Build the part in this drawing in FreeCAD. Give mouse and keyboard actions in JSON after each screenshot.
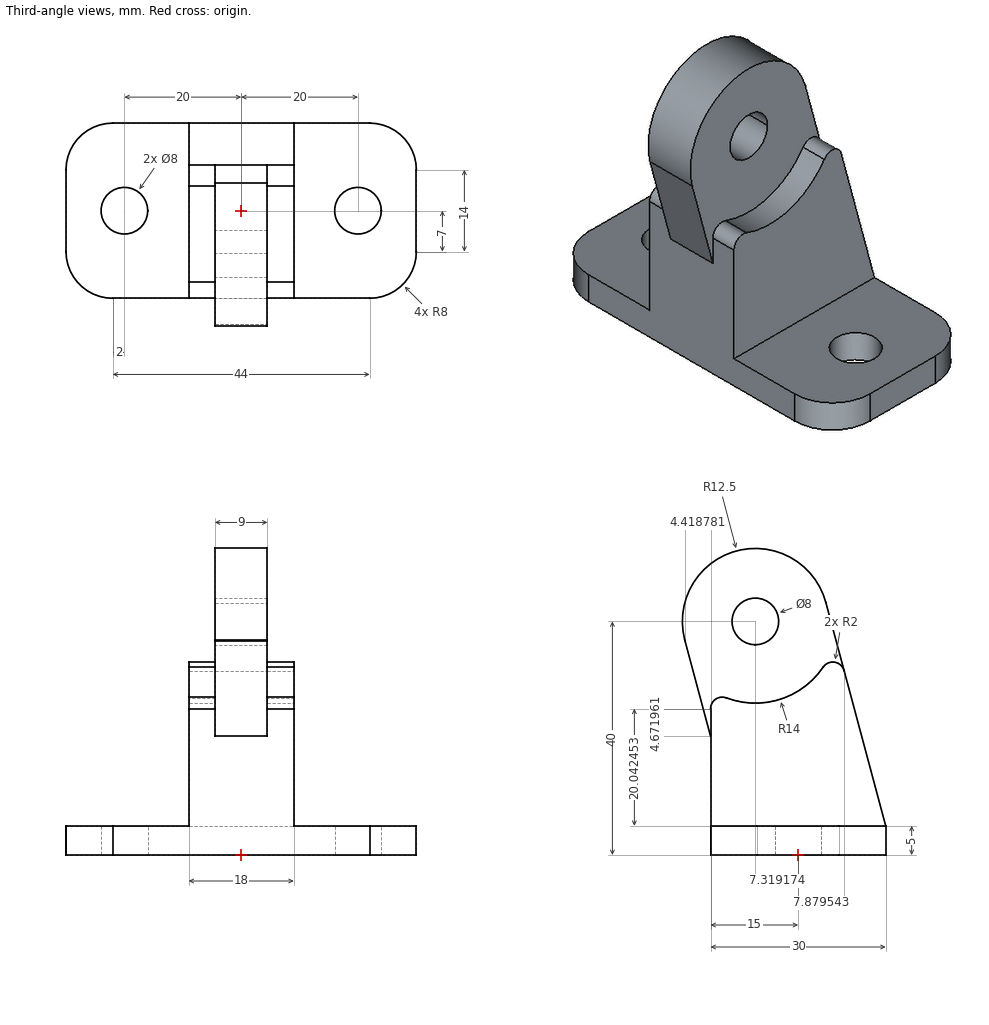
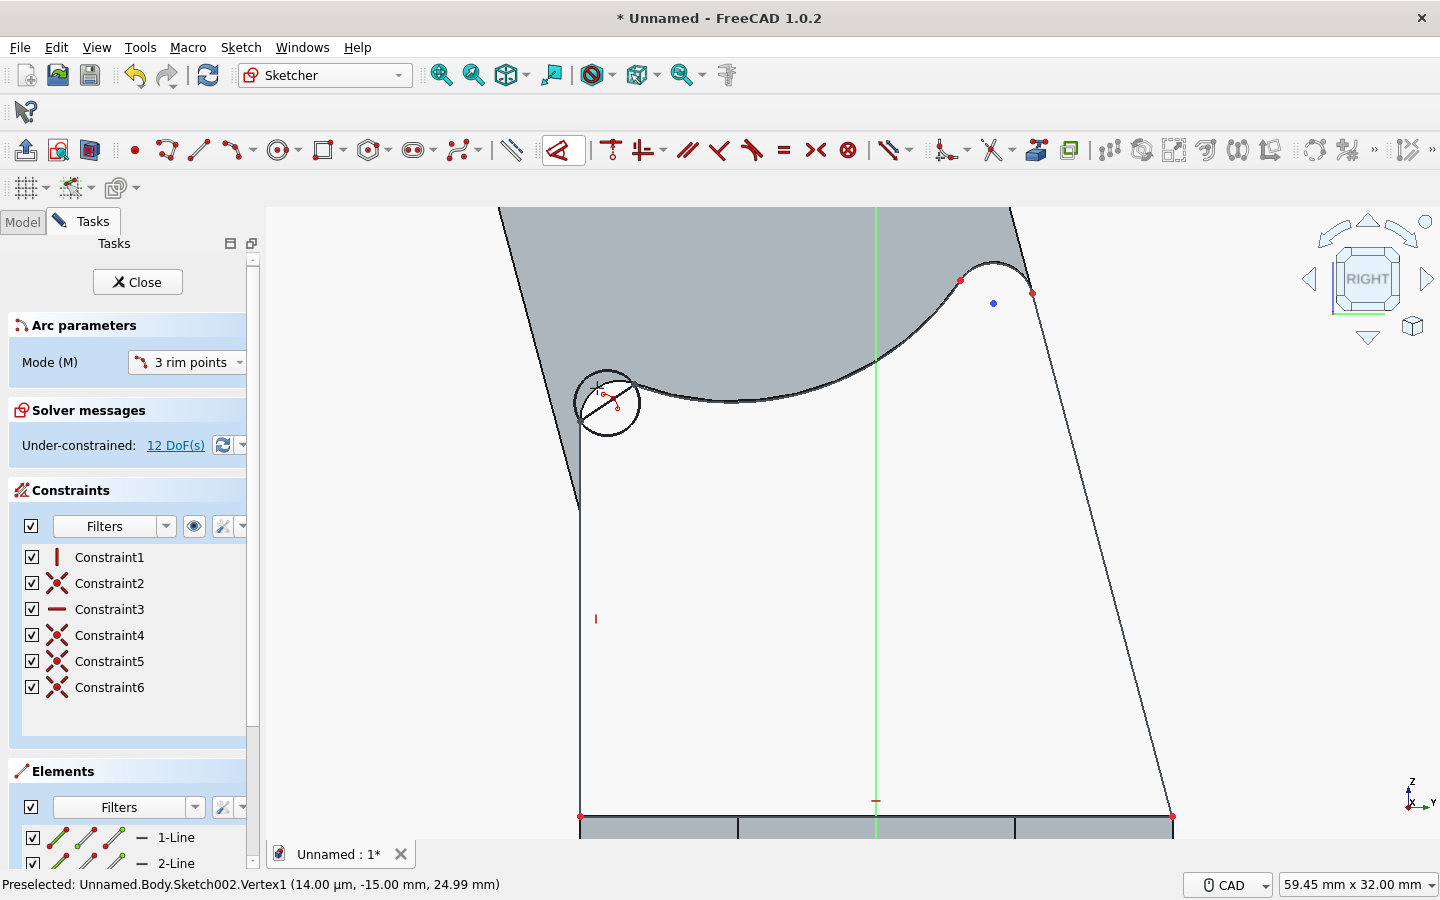
{"action": "left_click", "coordinate": [597, 388]}
{"action": "key", "text": "Escape"}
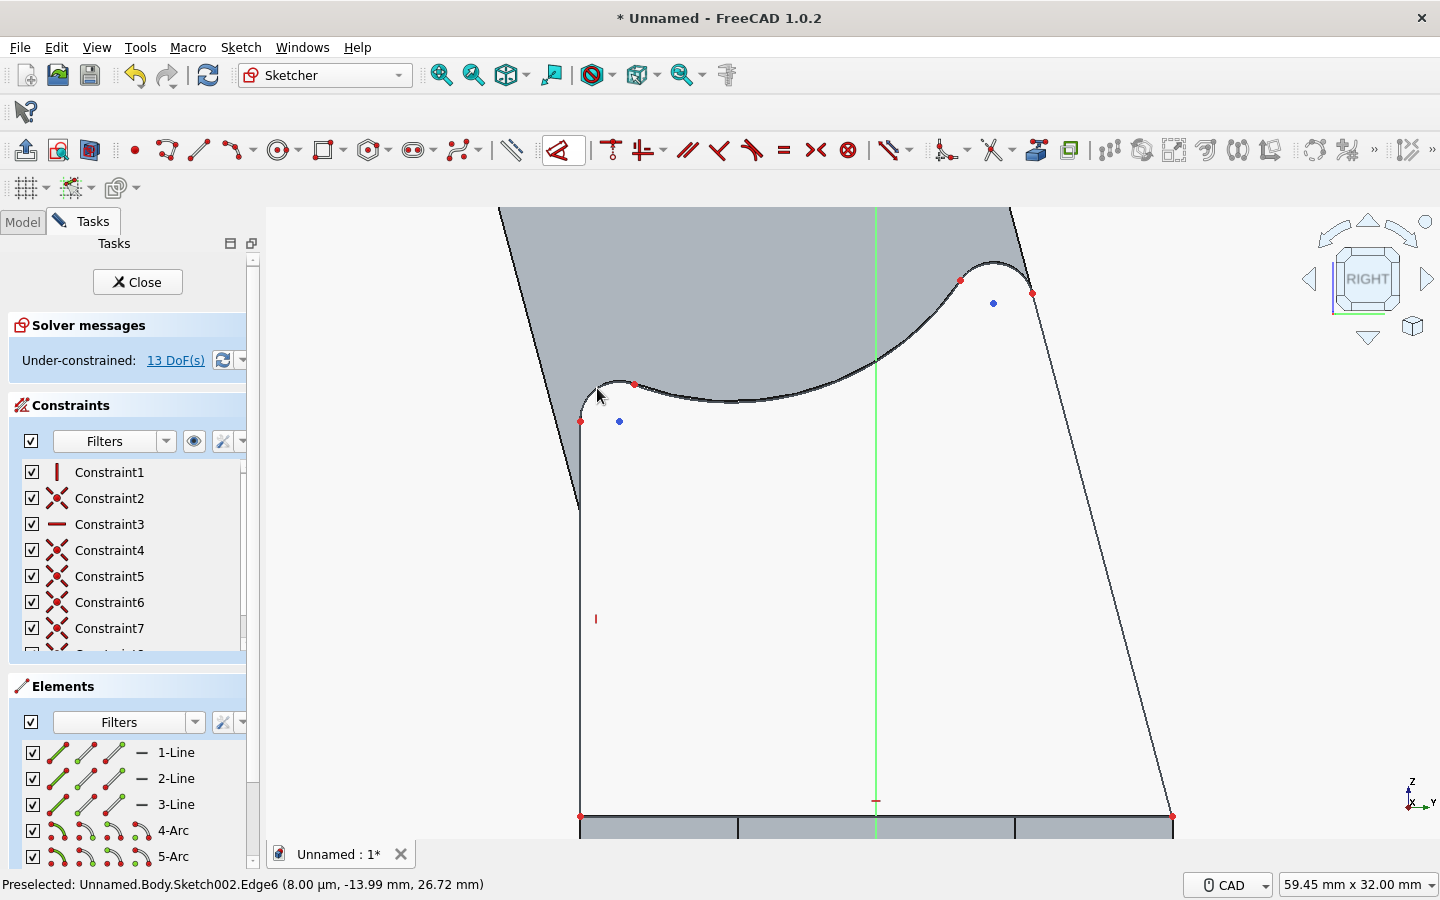
{"action": "left_click", "coordinate": [580, 540]}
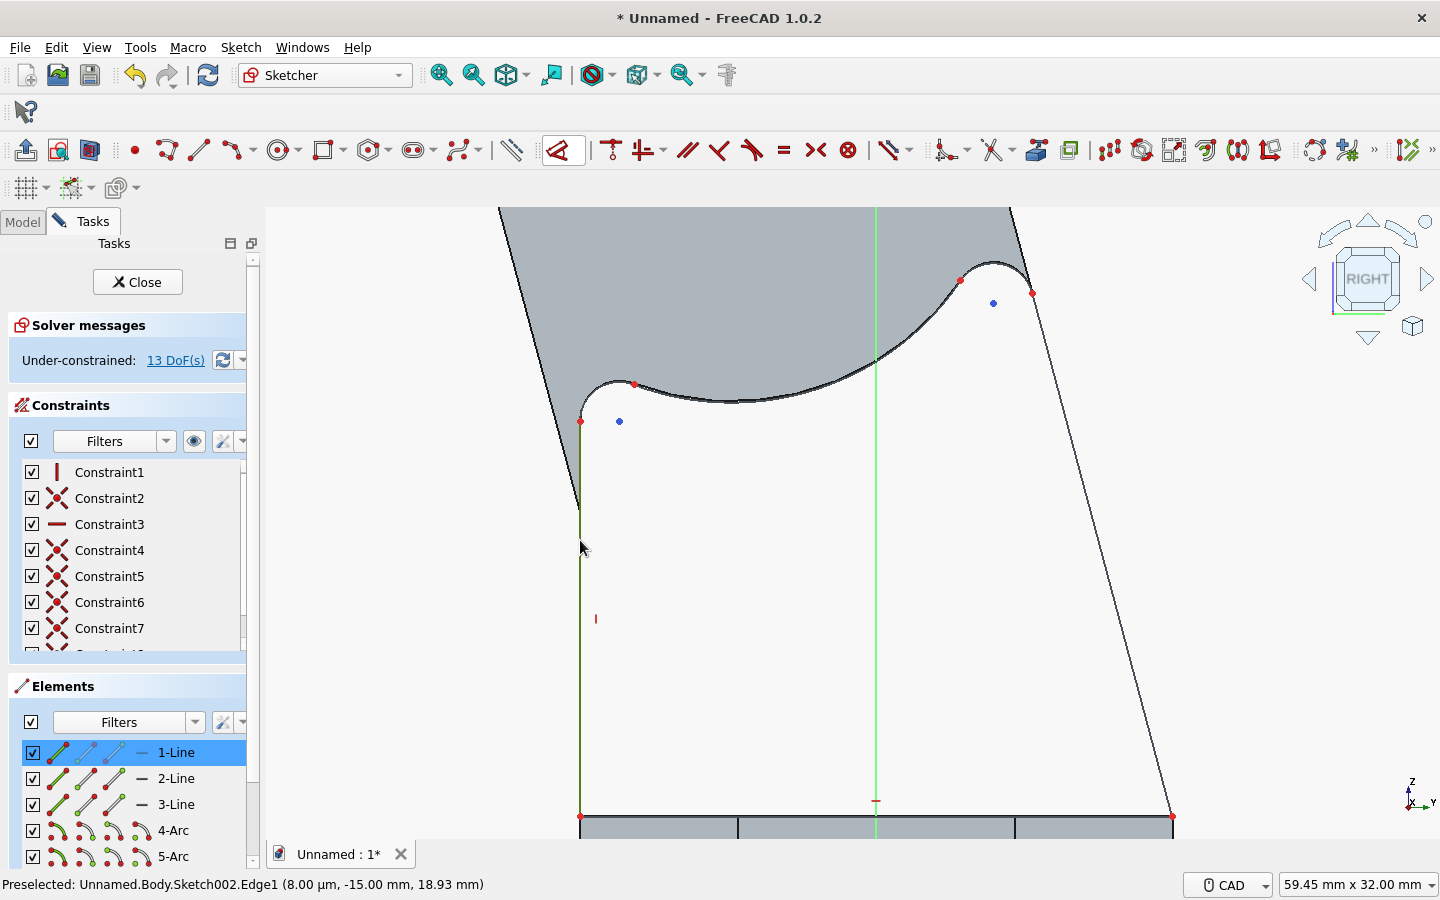
{"action": "left_click", "coordinate": [612, 383]}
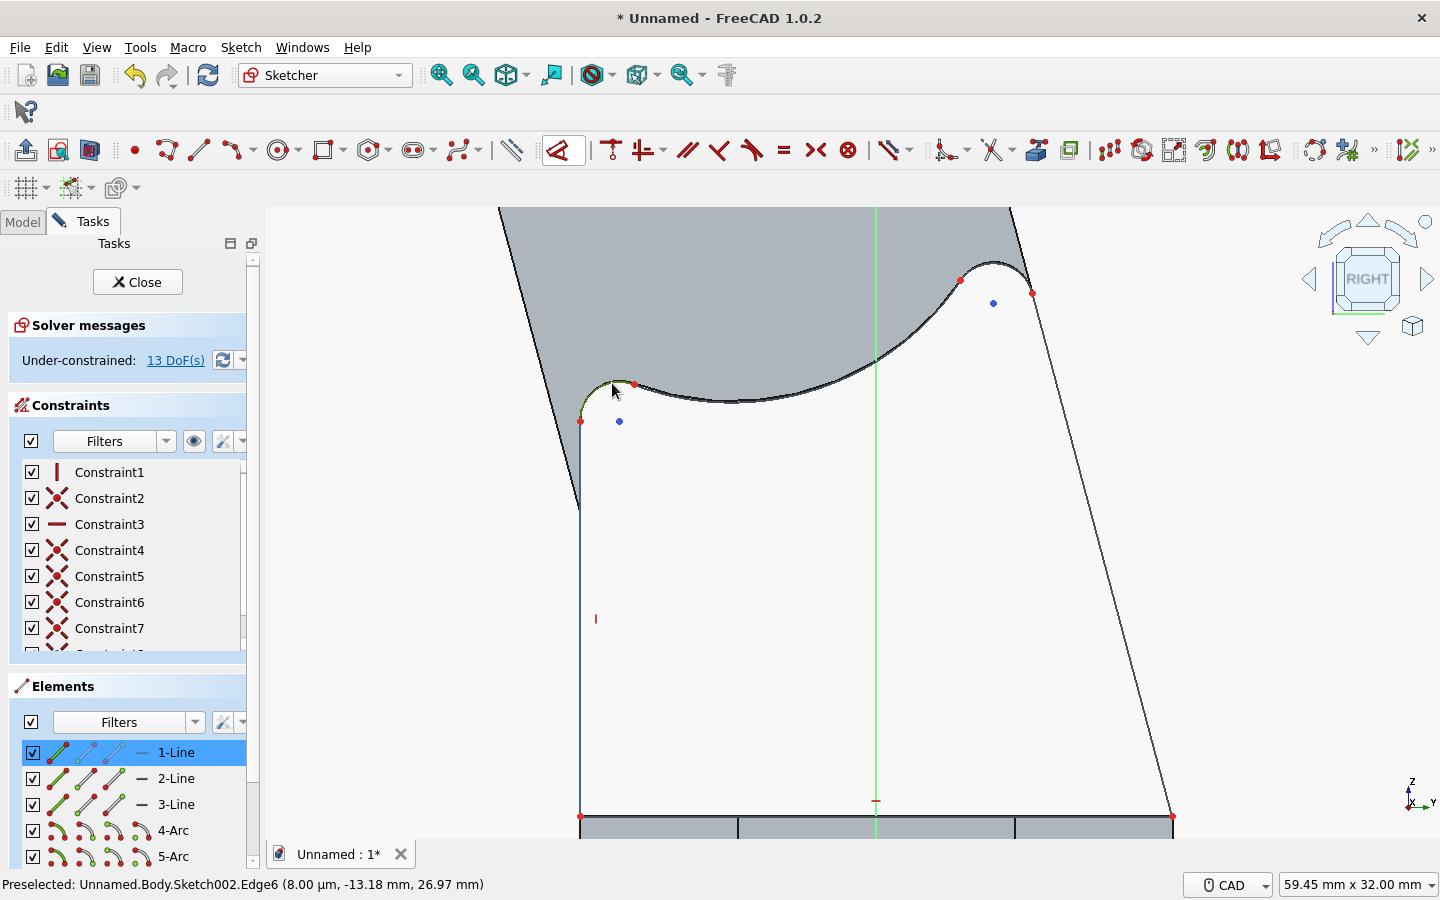
{"action": "left_click", "coordinate": [752, 150]}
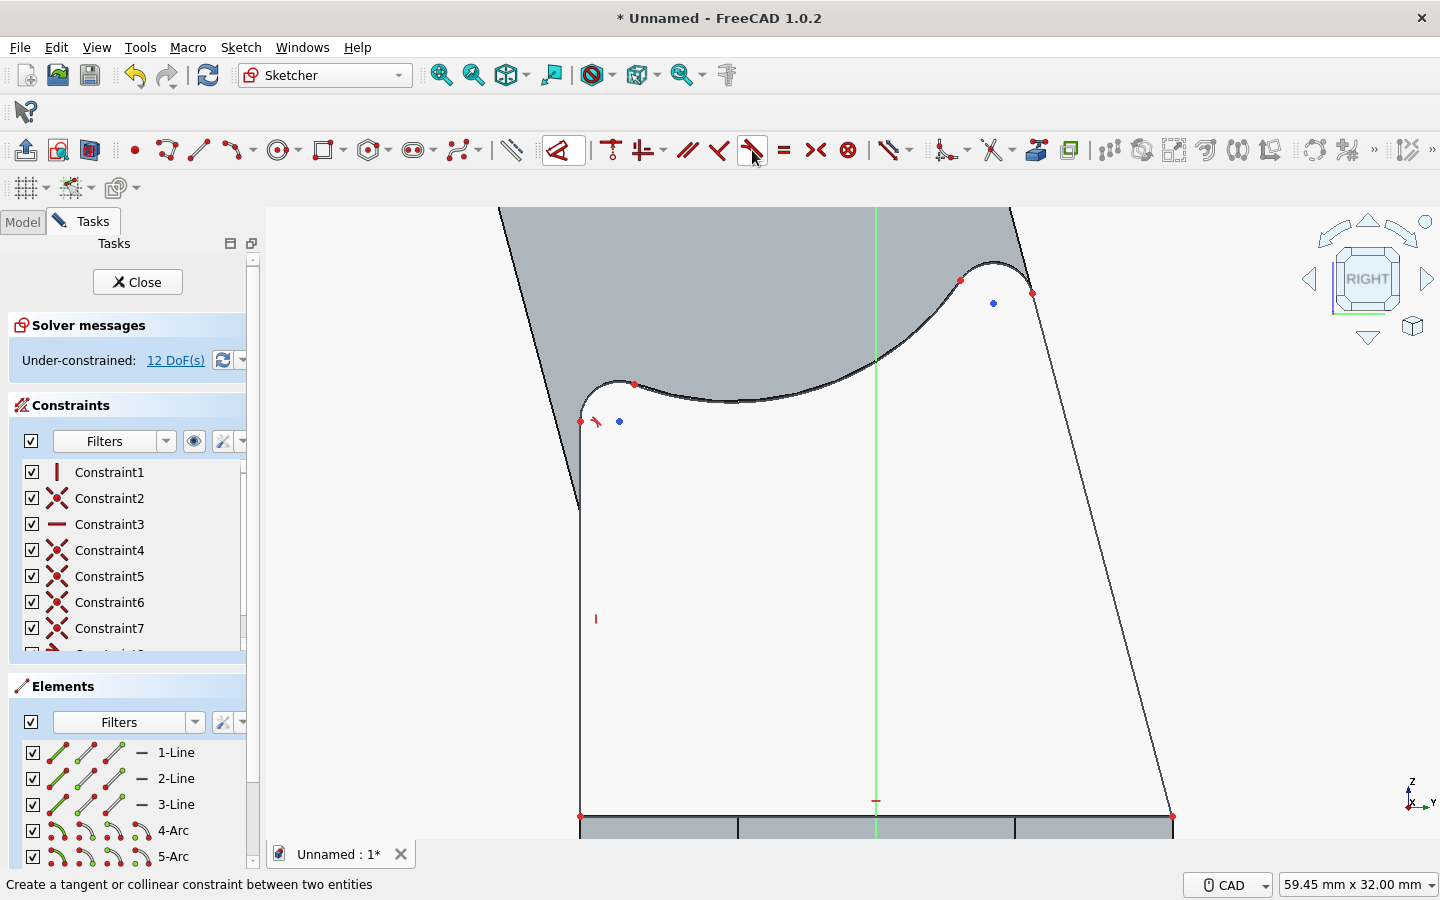
{"action": "left_click", "coordinate": [1130, 660]}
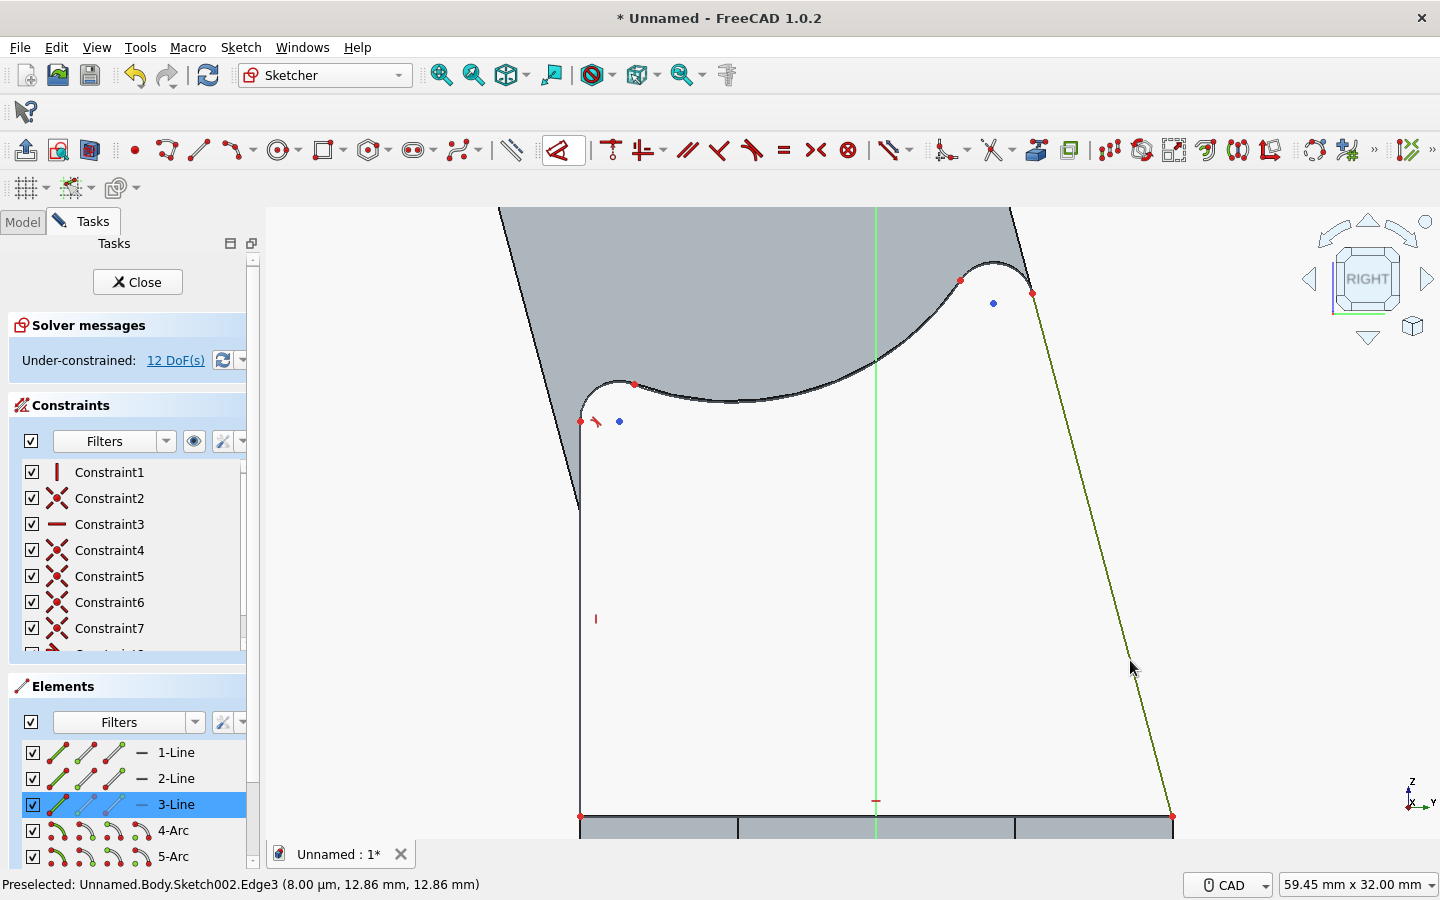
{"action": "left_click", "coordinate": [1017, 271]}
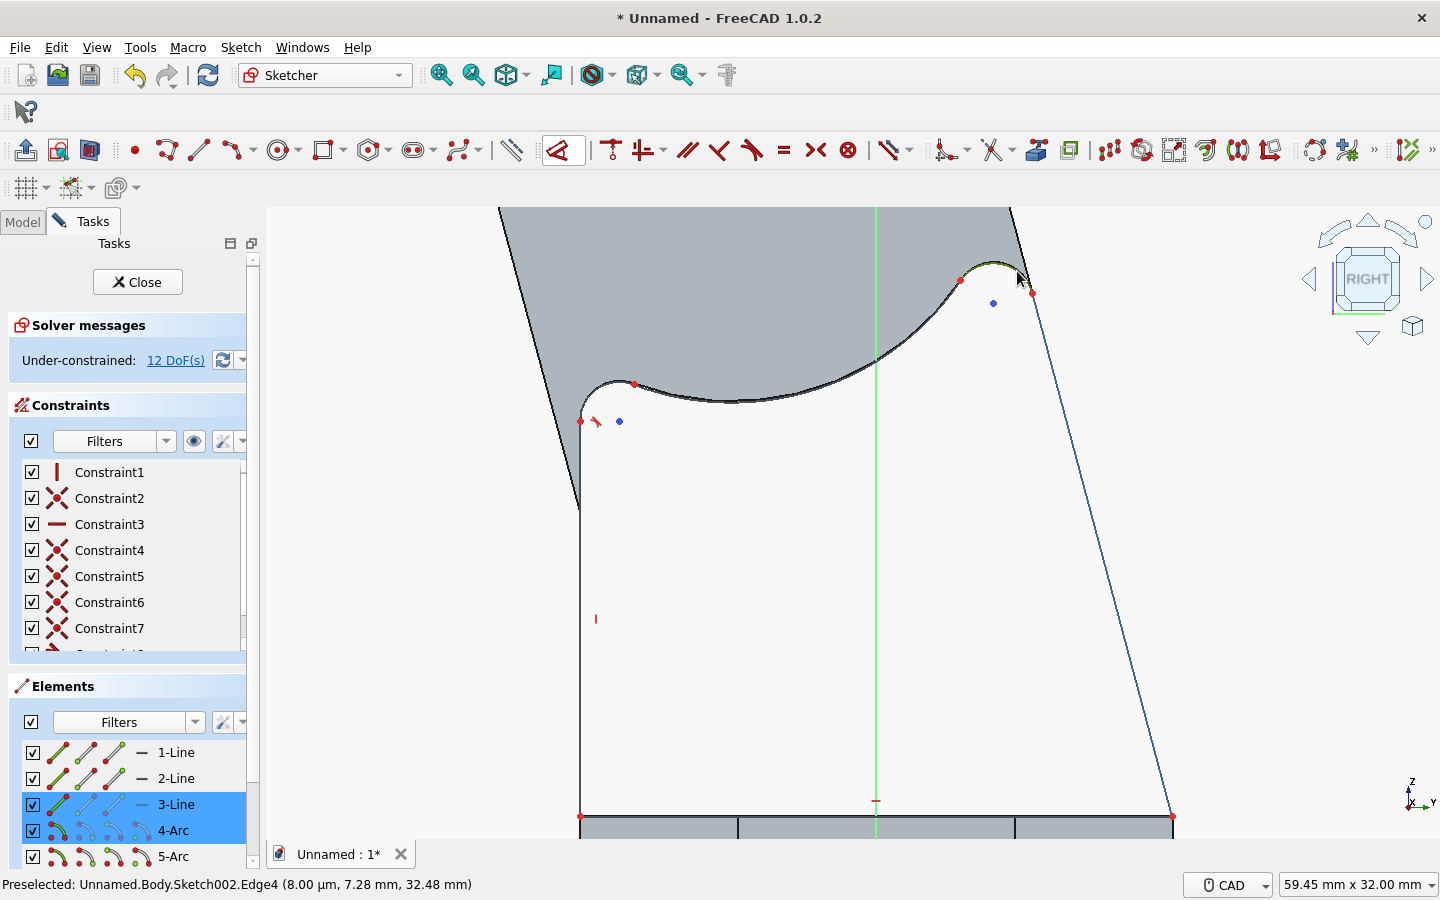
{"action": "key", "text": "t"}